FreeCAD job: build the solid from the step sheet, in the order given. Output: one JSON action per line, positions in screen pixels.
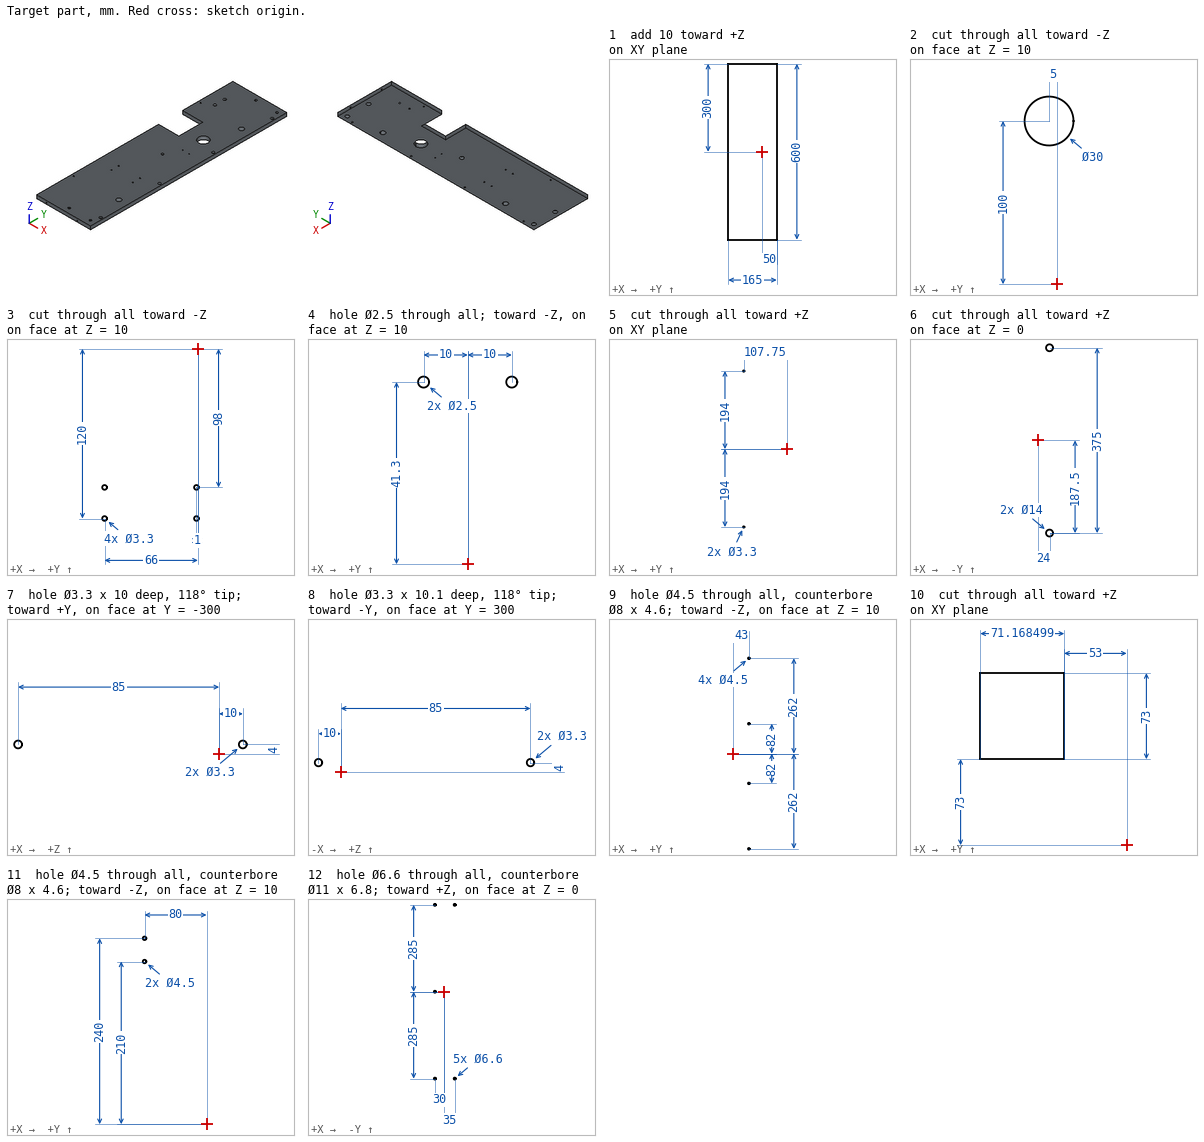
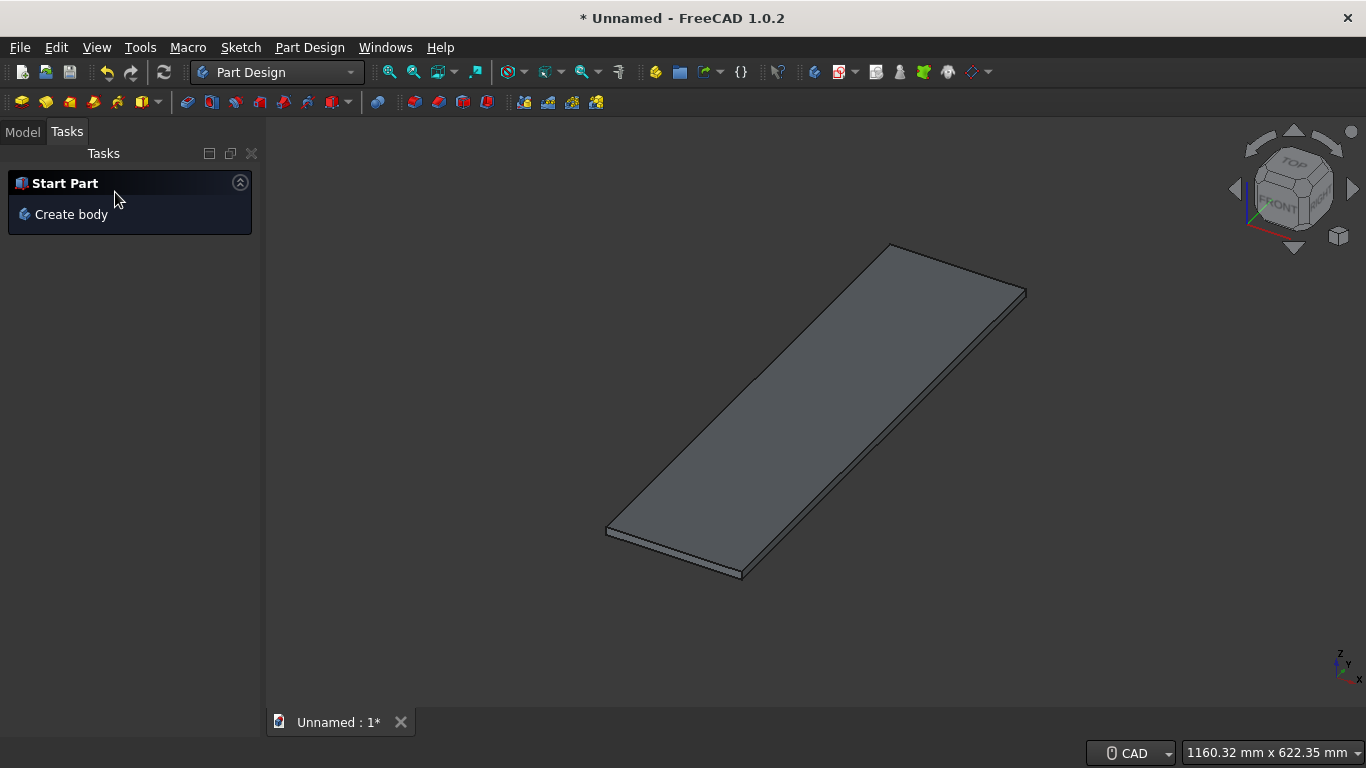
{"action": "left_click", "coordinate": [897, 326]}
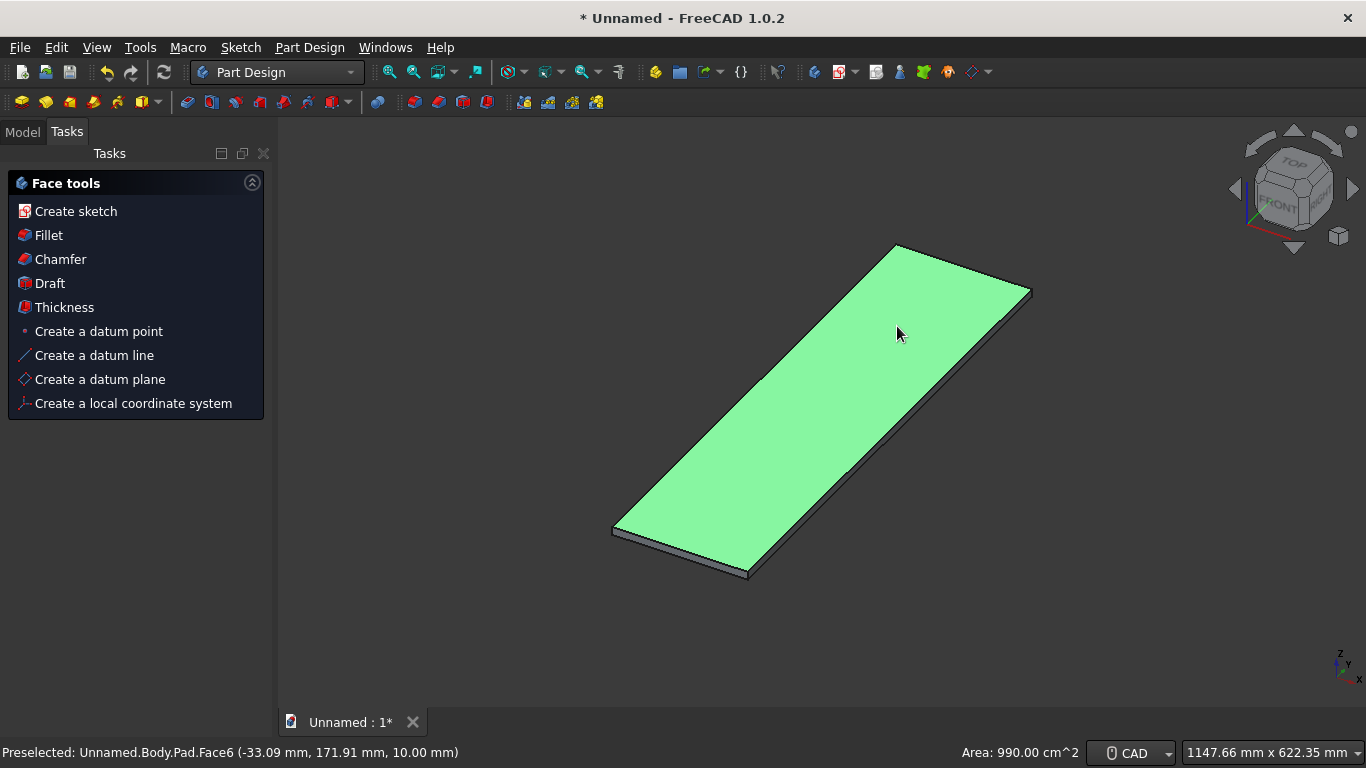
{"action": "left_click", "coordinate": [840, 72]}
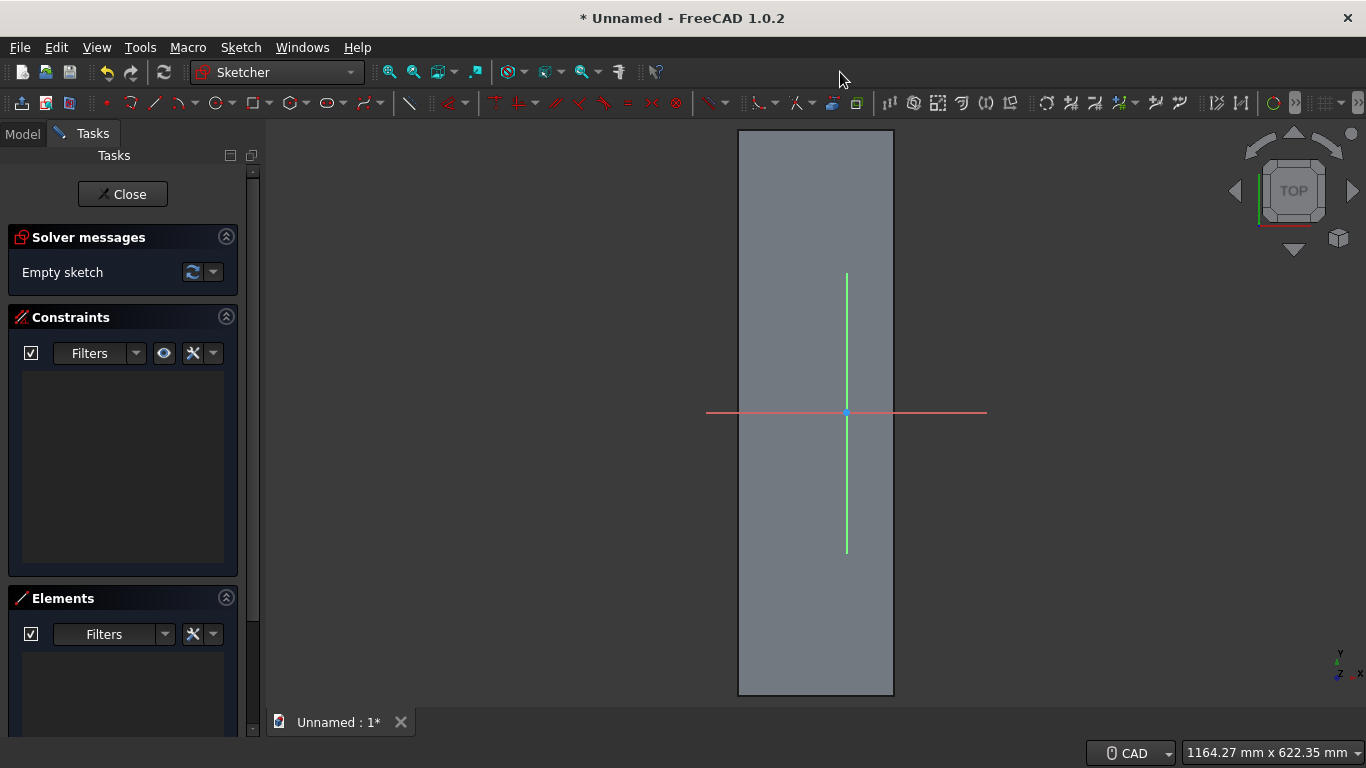
{"action": "scroll", "coordinate": [850, 311], "scroll_direction": "up", "scroll_amount": 13}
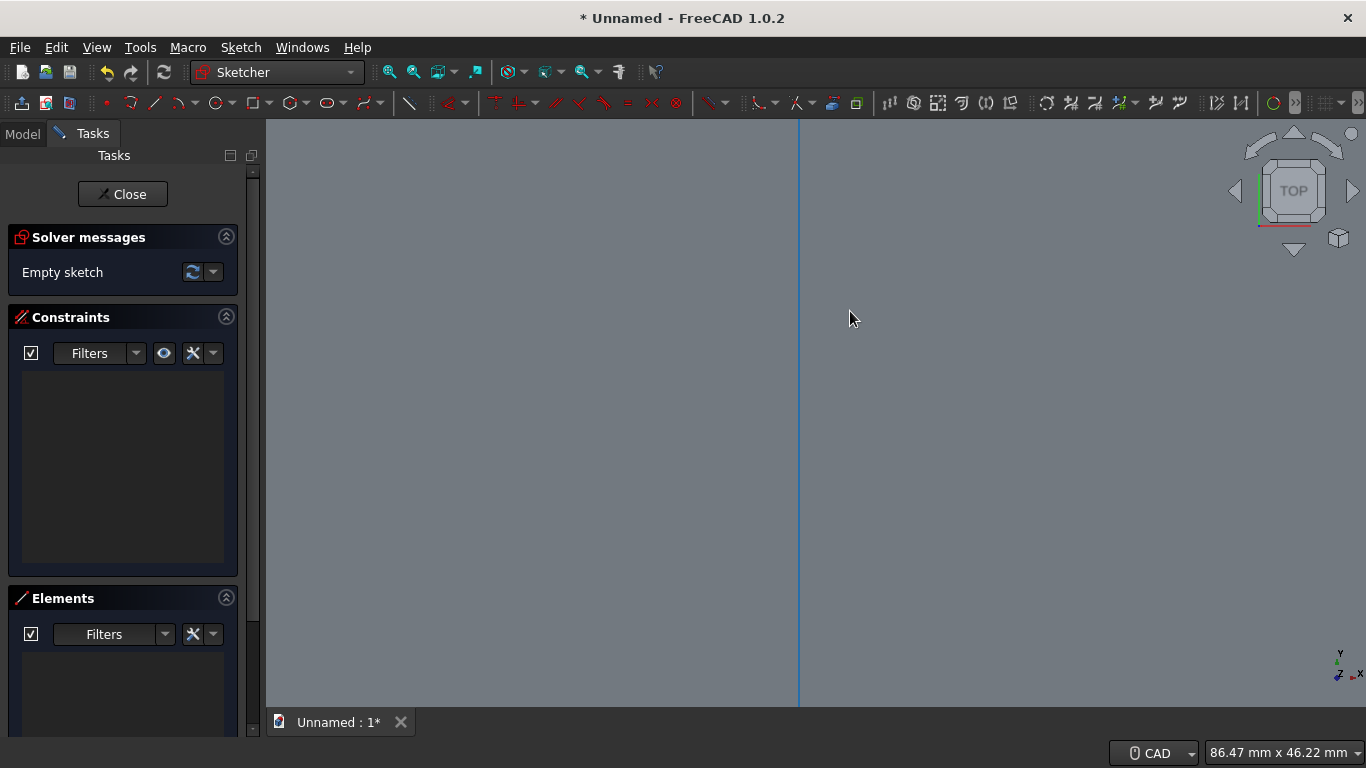
{"action": "left_click", "coordinate": [216, 104]}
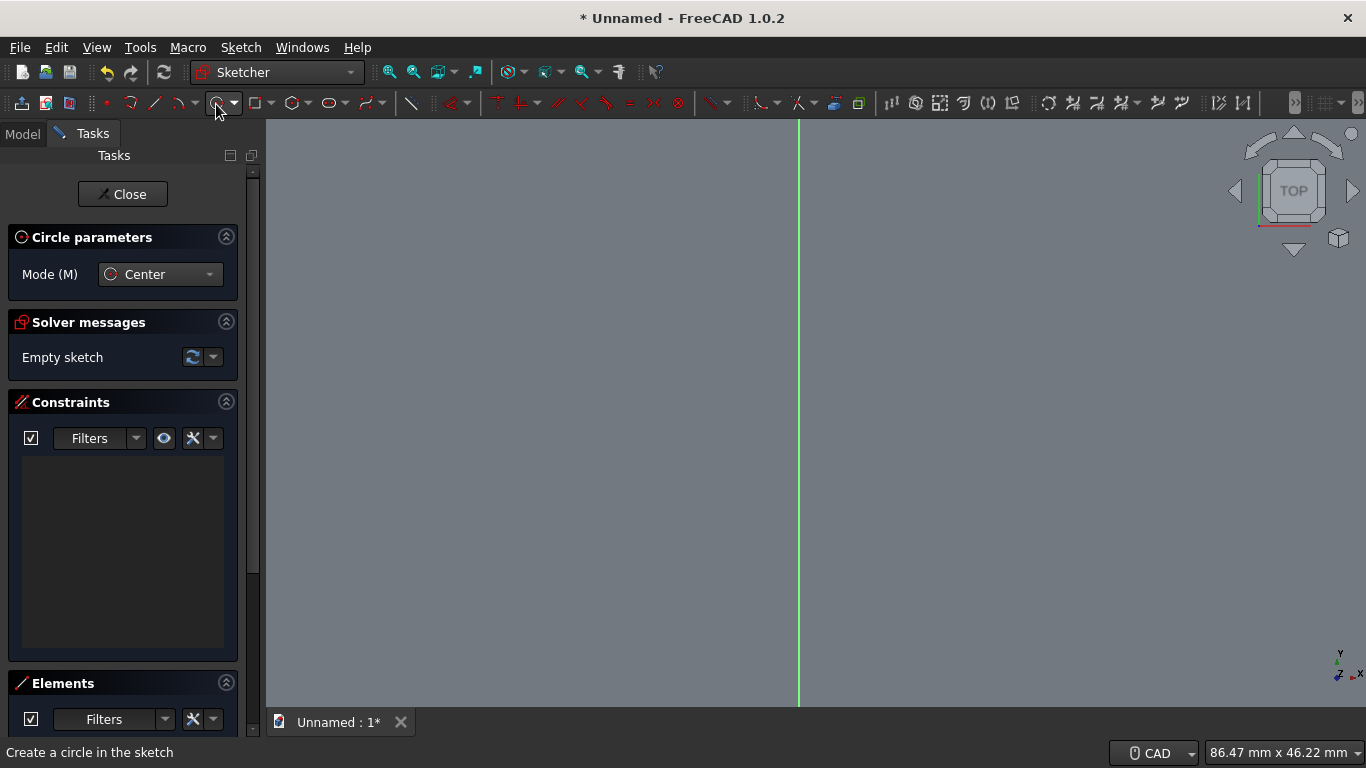
{"action": "left_click", "coordinate": [735, 408]}
{"action": "mouse_move", "coordinate": [870, 273]}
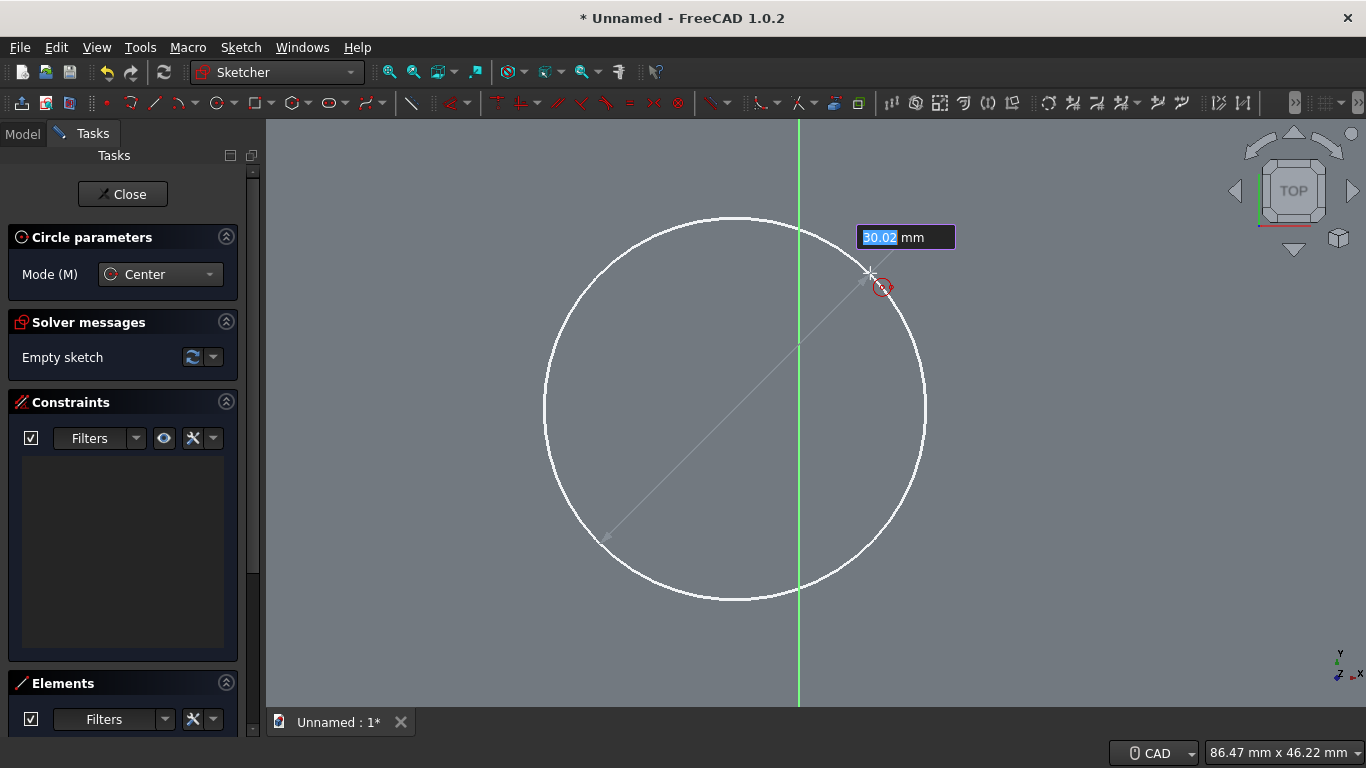
{"action": "type", "text": "30"}
{"action": "key", "text": "Return"}
{"action": "key", "text": "Escape"}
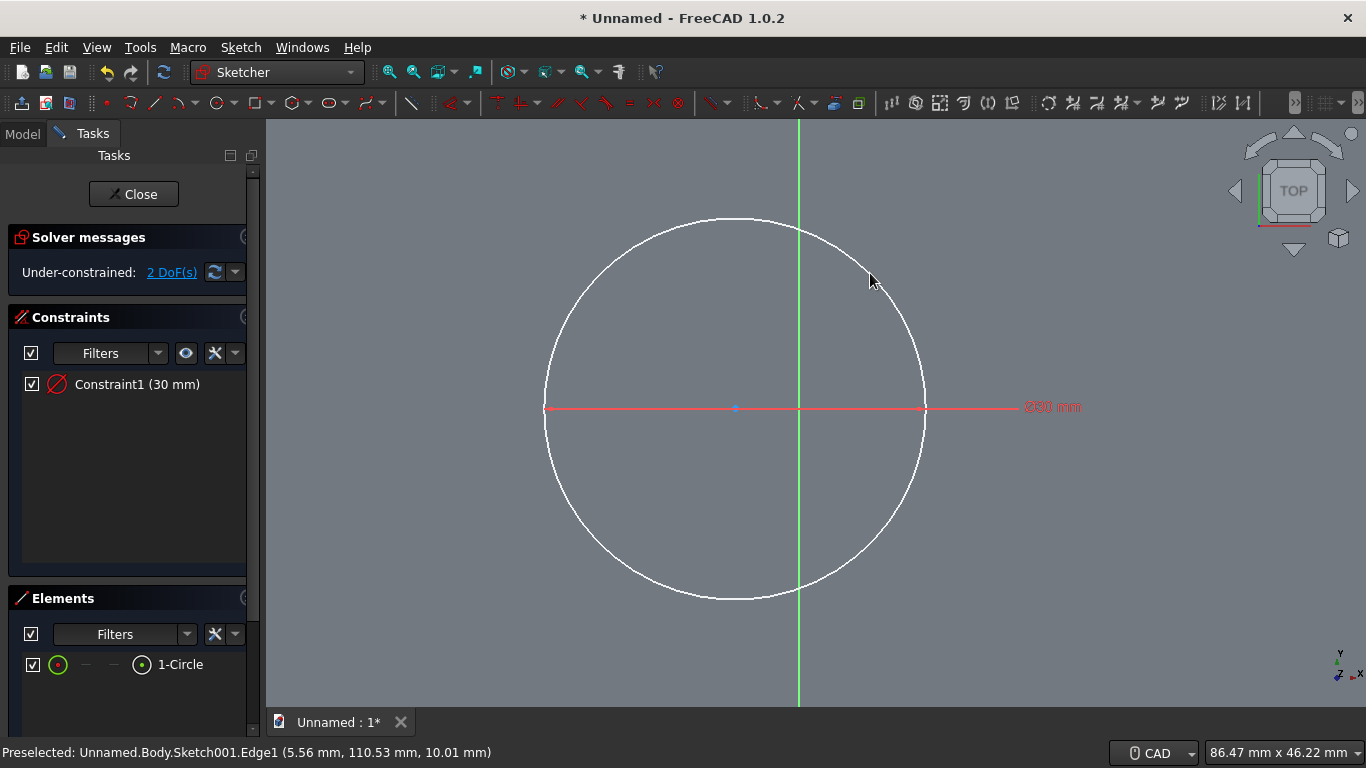
{"action": "key", "text": "d"}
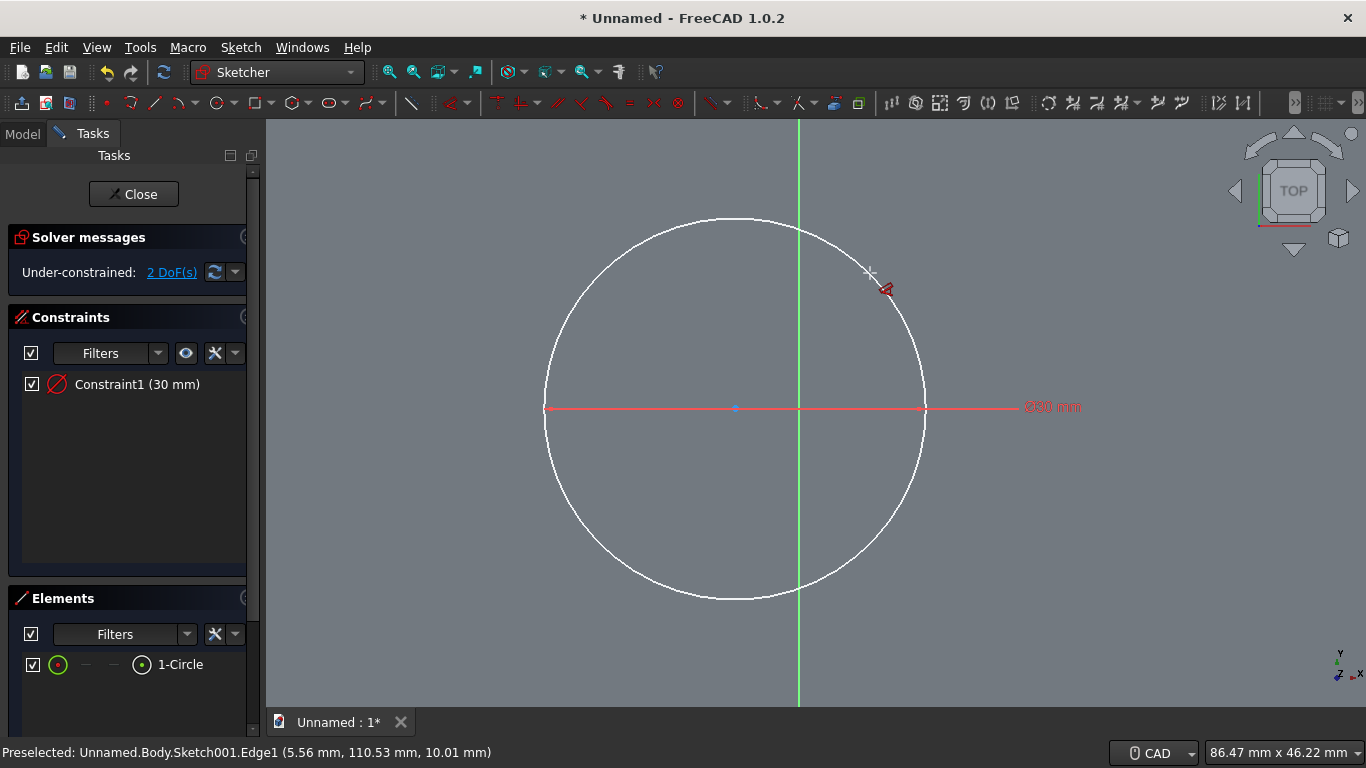
{"action": "left_click", "coordinate": [735, 409]}
{"action": "left_click", "coordinate": [767, 375]}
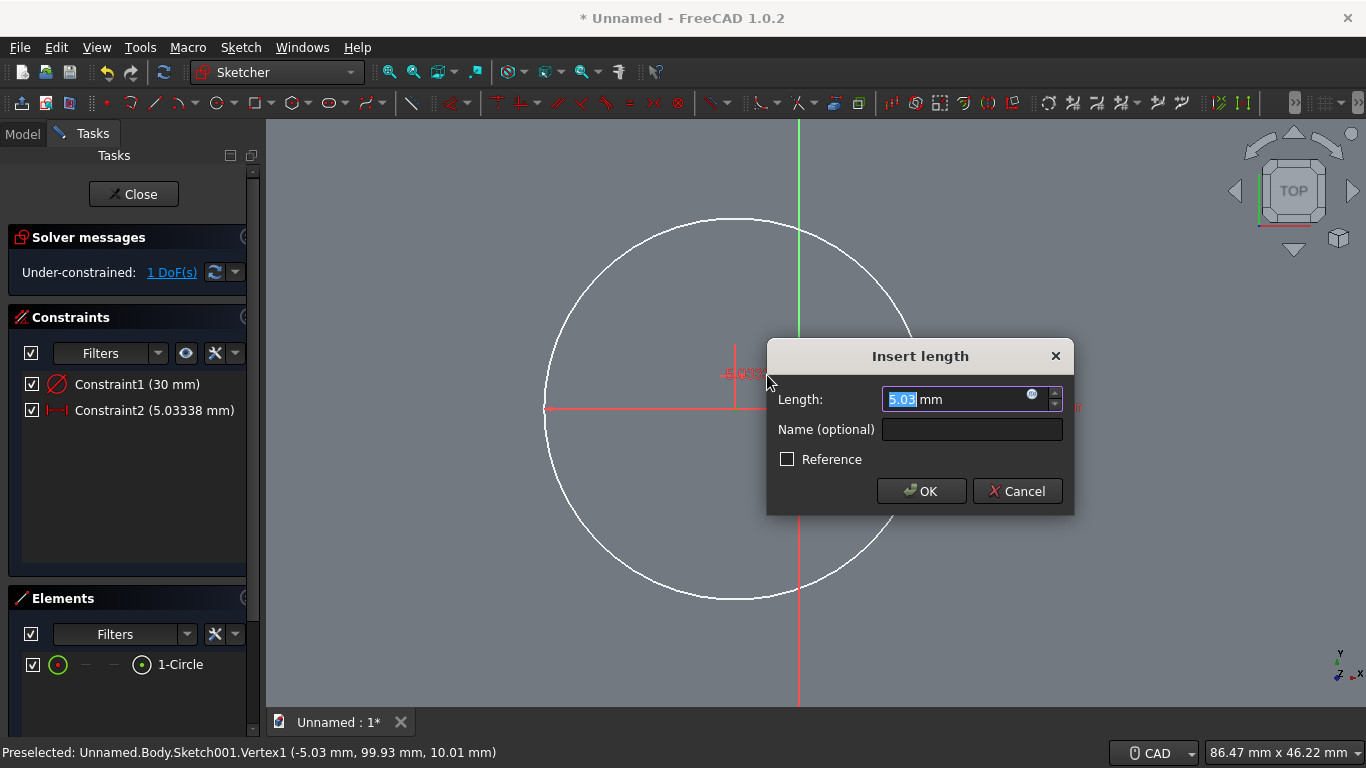
{"action": "type", "text": "5"}
{"action": "key", "text": "Return"}